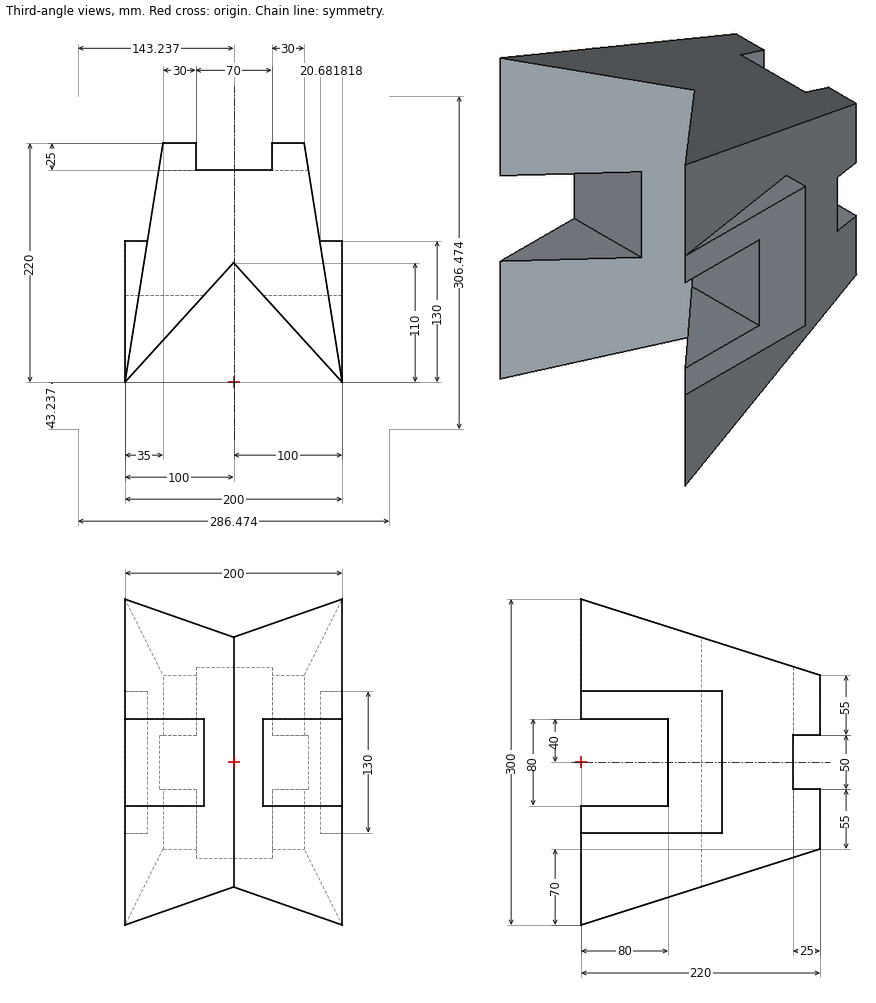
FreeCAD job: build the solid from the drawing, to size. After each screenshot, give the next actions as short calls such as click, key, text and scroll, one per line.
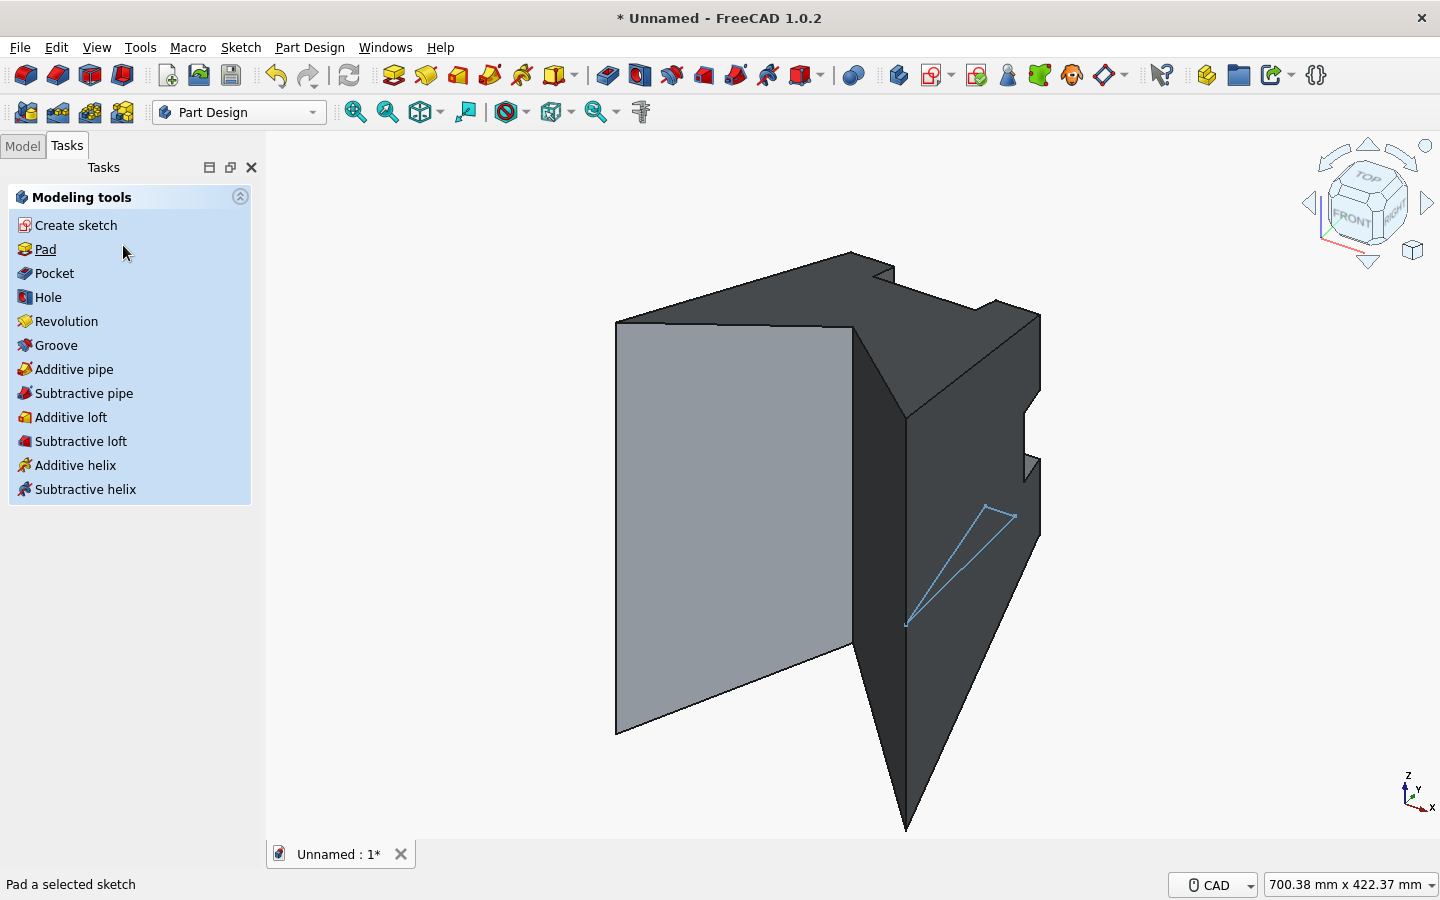
click(394, 76)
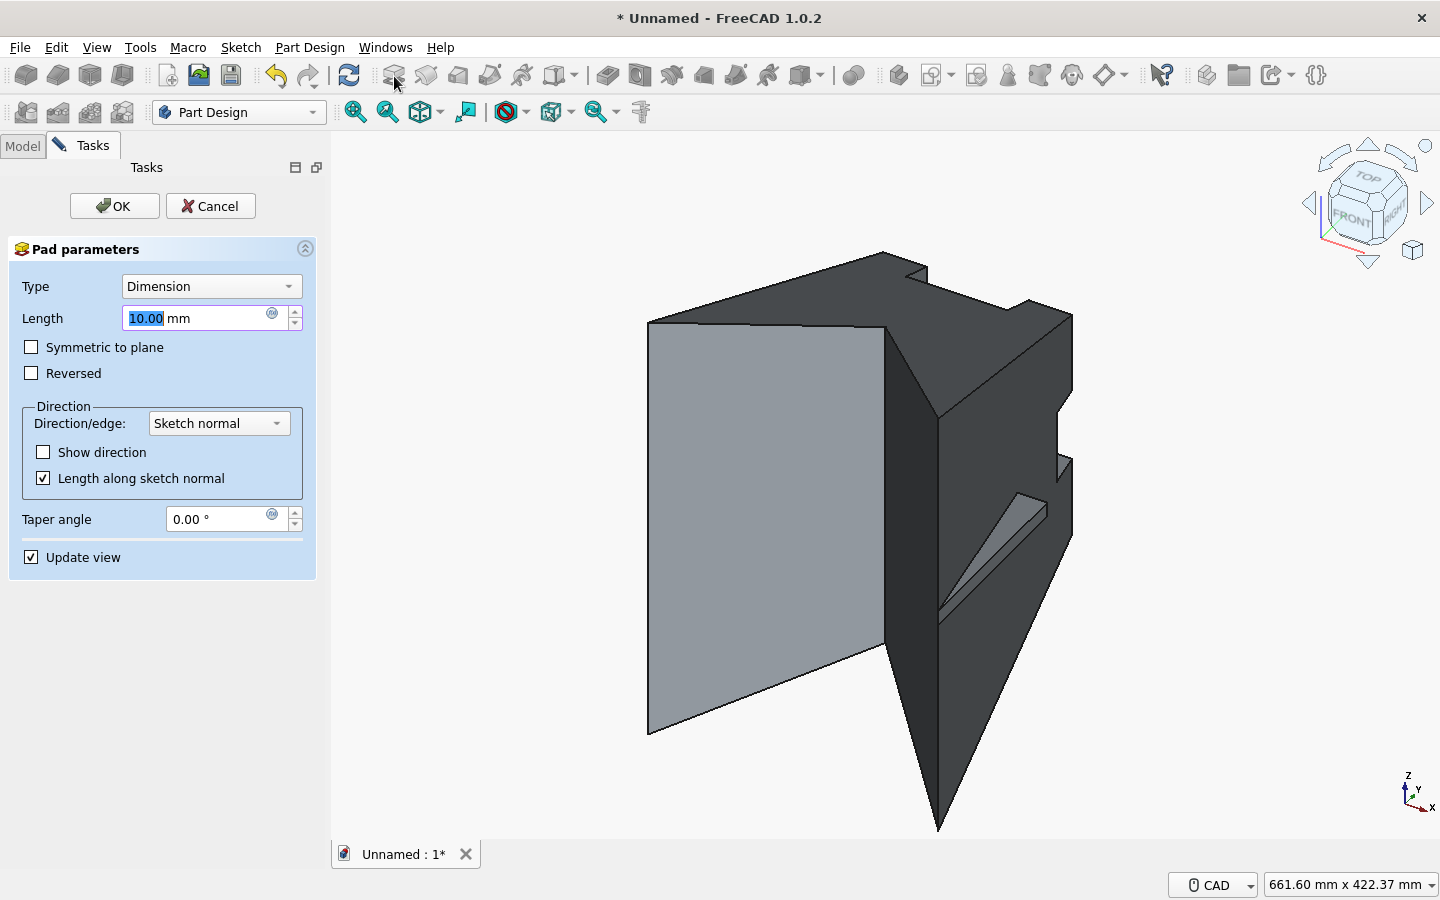
text(130)
key(Tab)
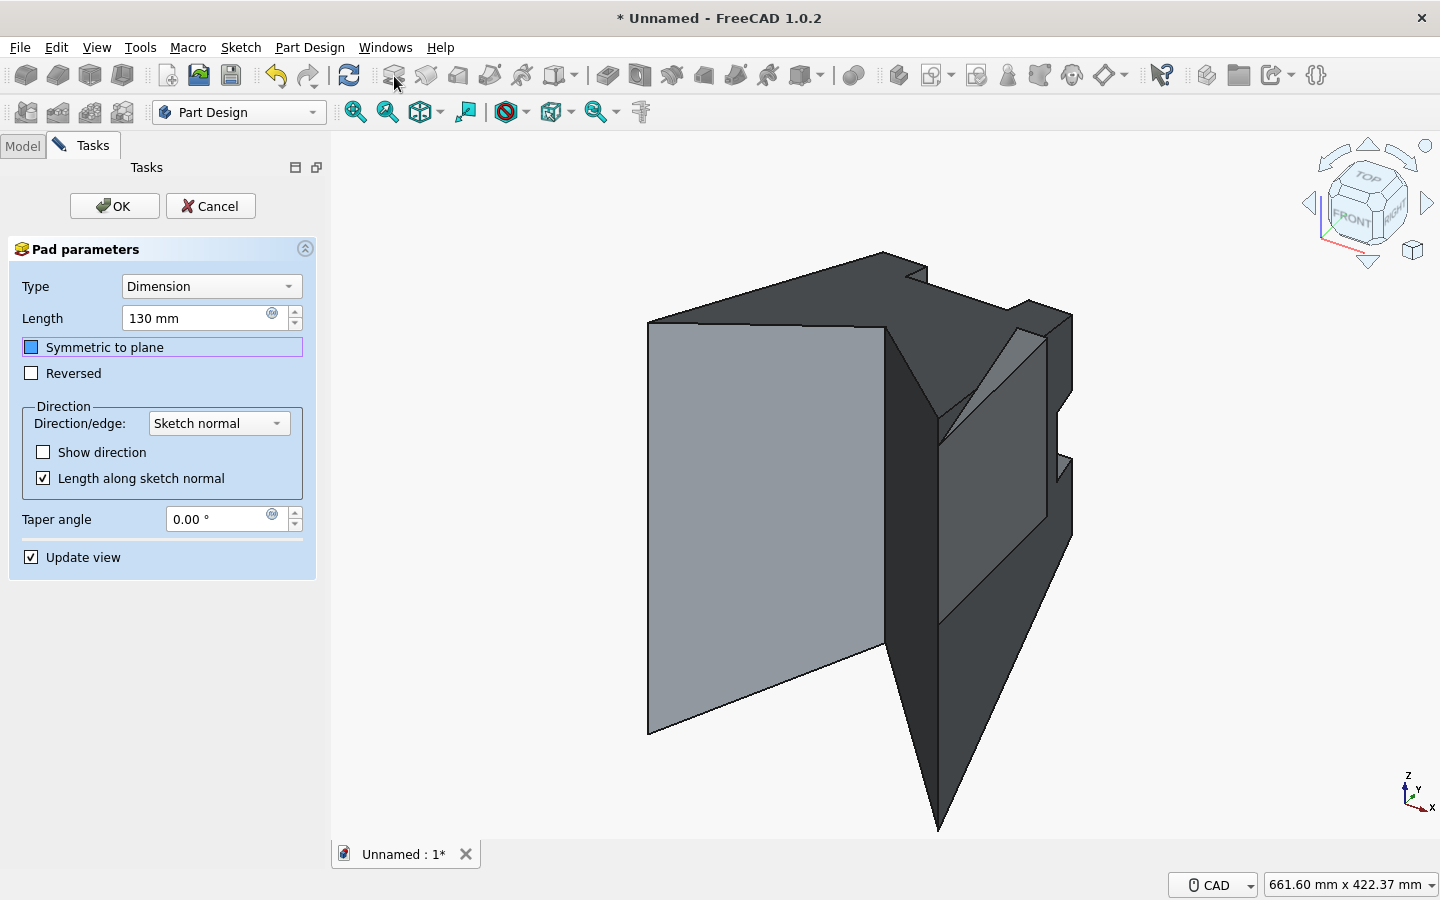
click(30, 347)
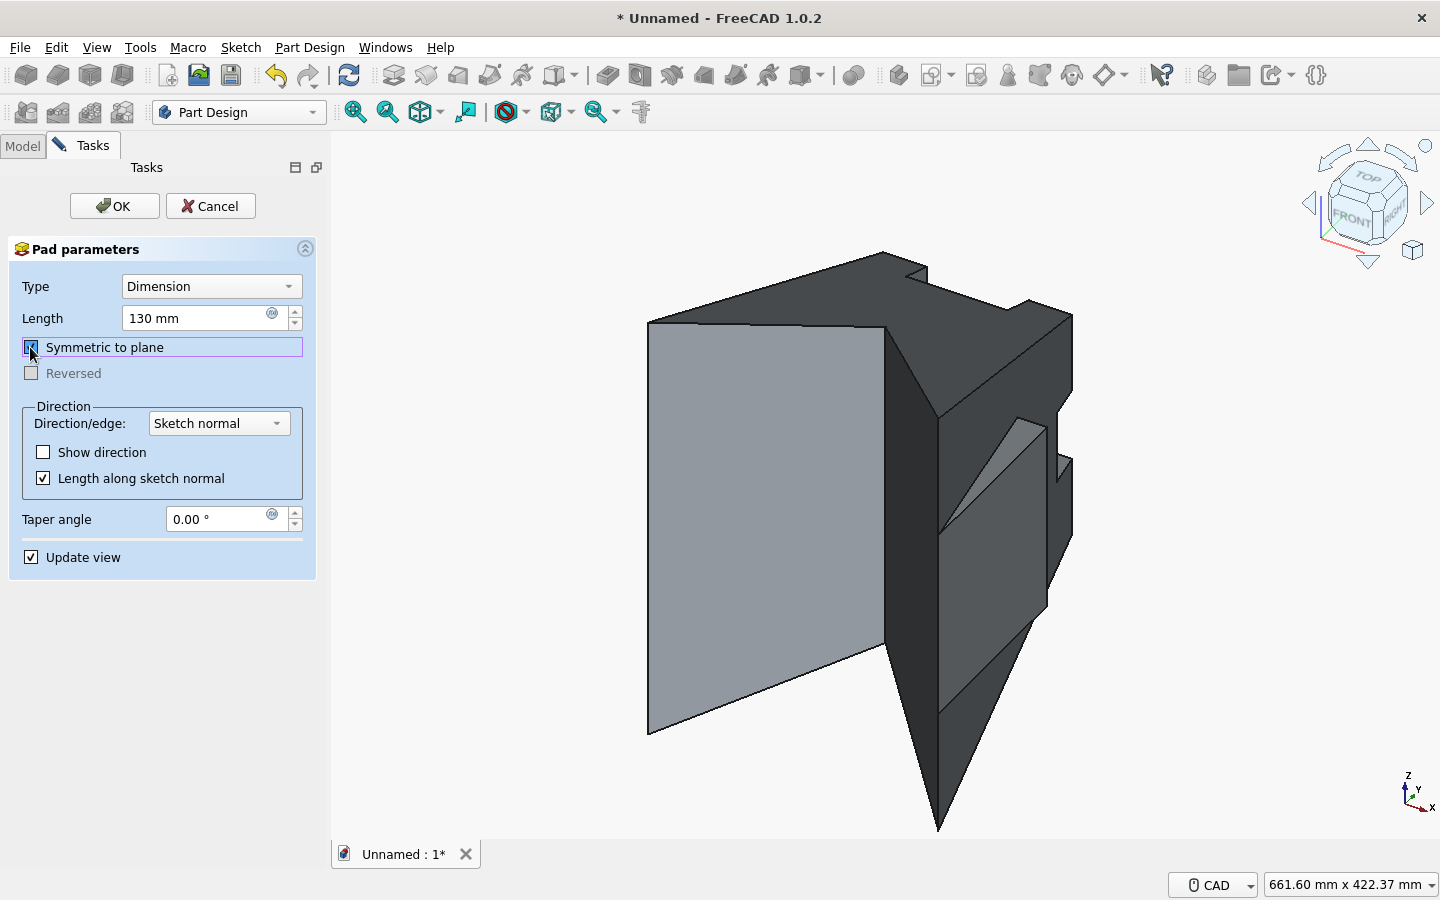
click(115, 206)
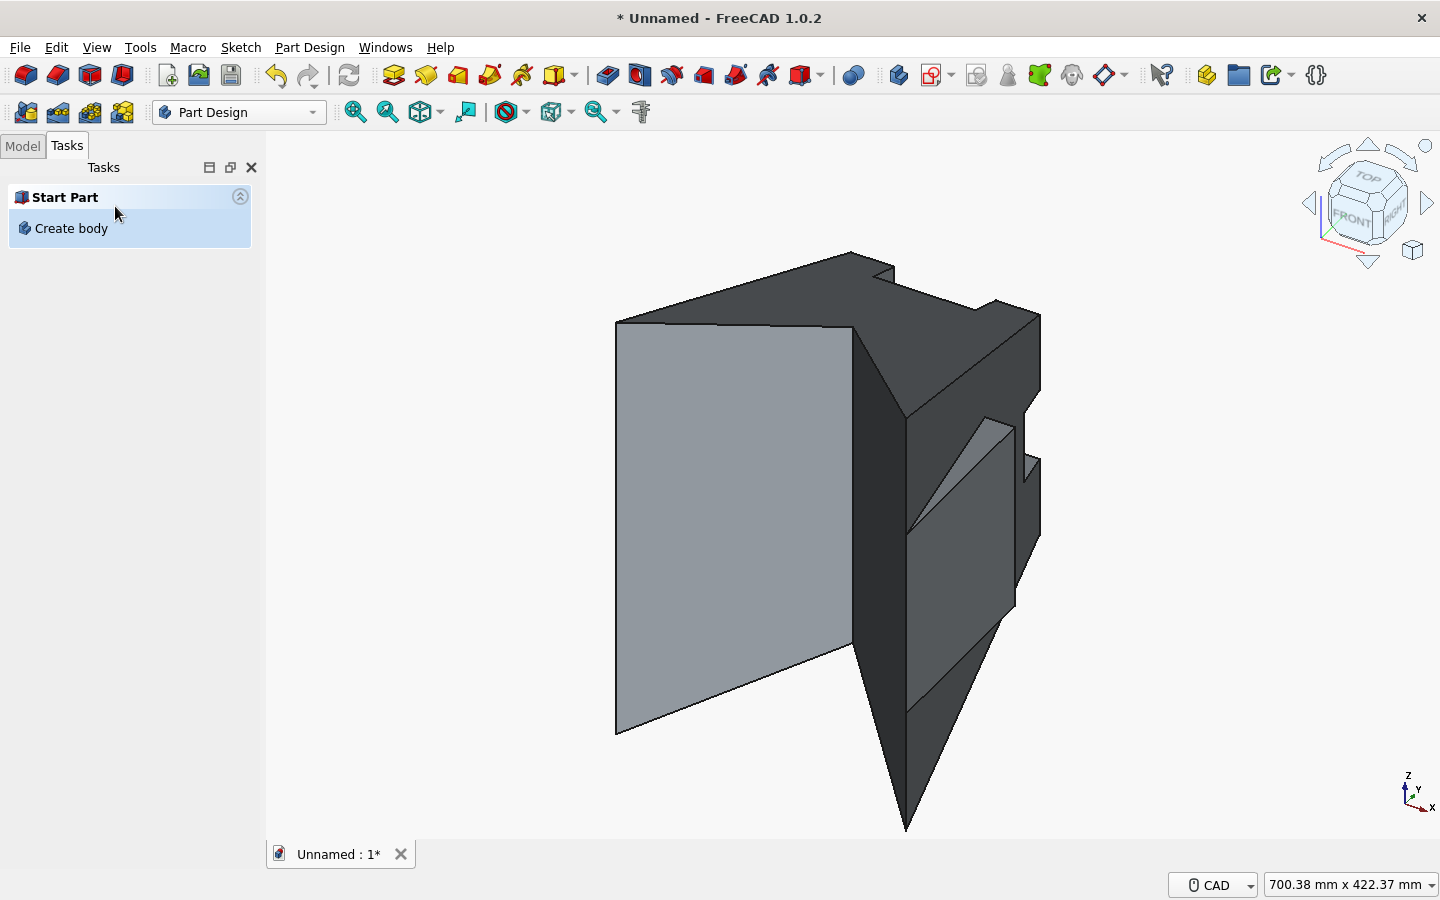
click(23, 145)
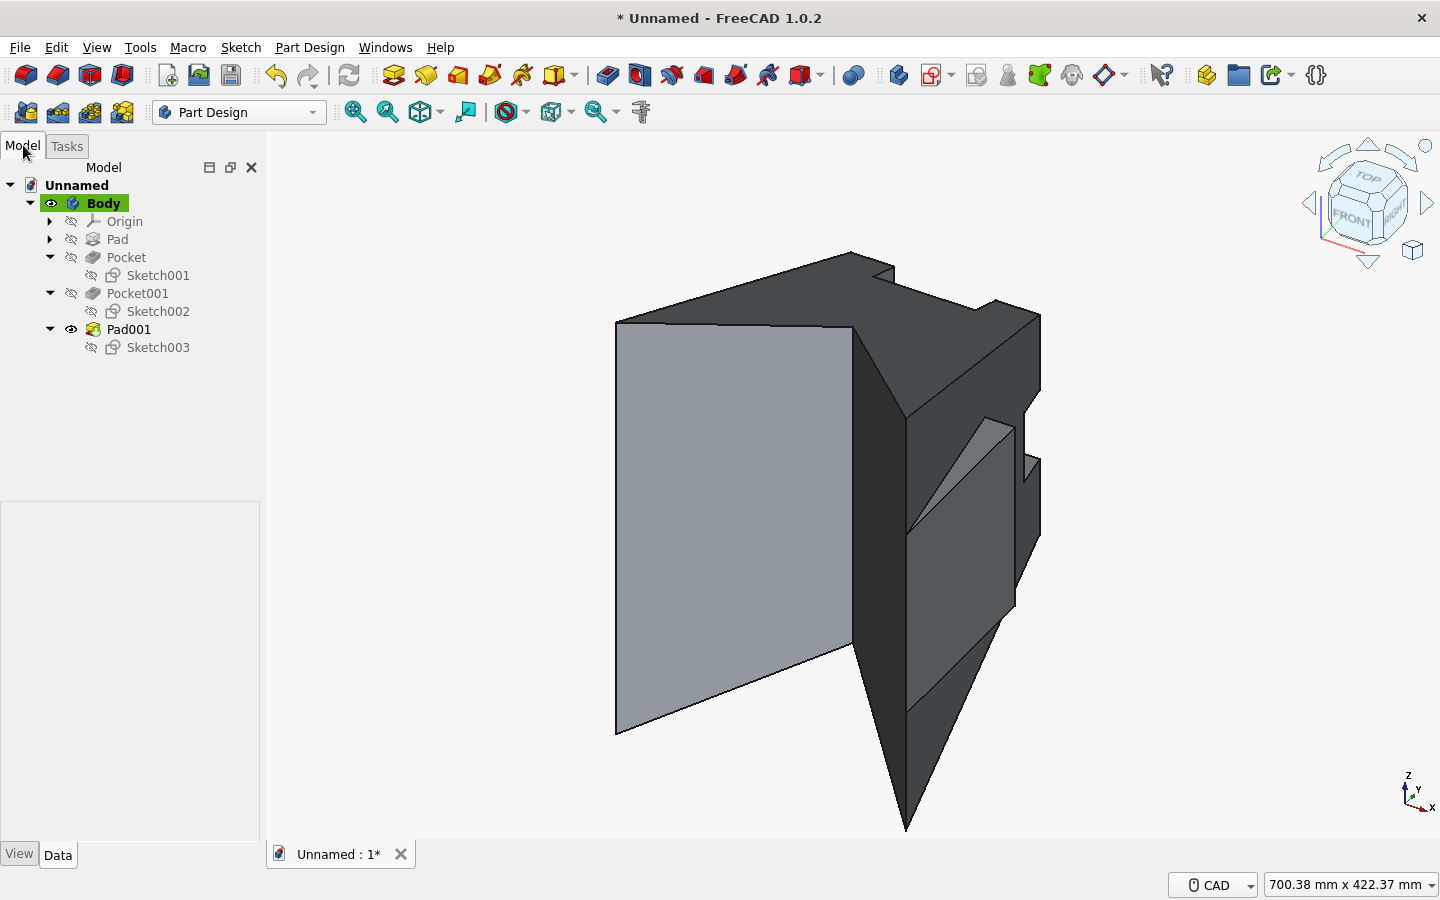
click(116, 329)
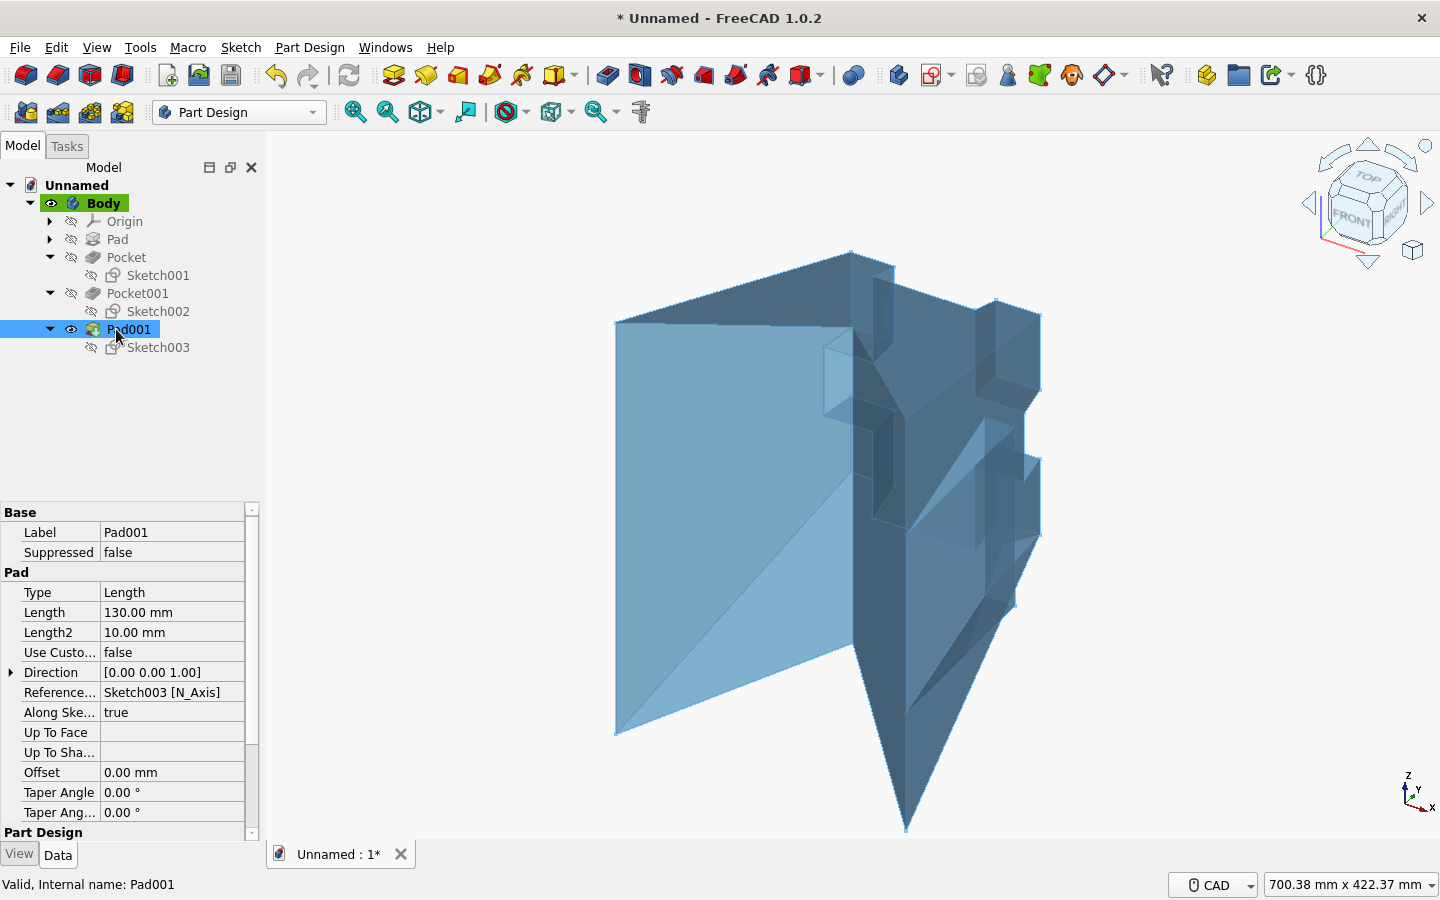
click(26, 112)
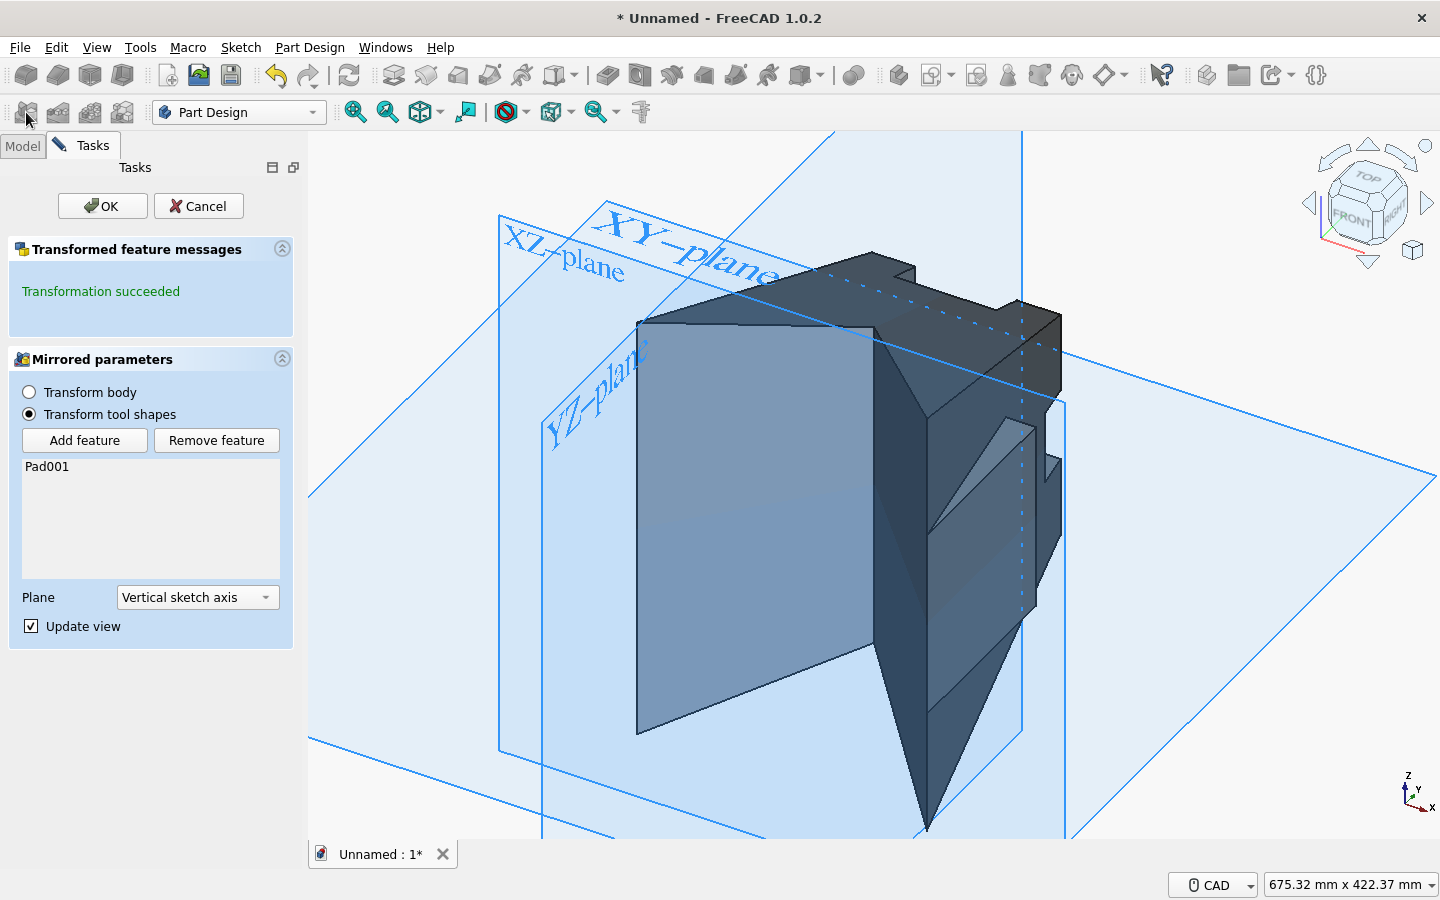
click(198, 598)